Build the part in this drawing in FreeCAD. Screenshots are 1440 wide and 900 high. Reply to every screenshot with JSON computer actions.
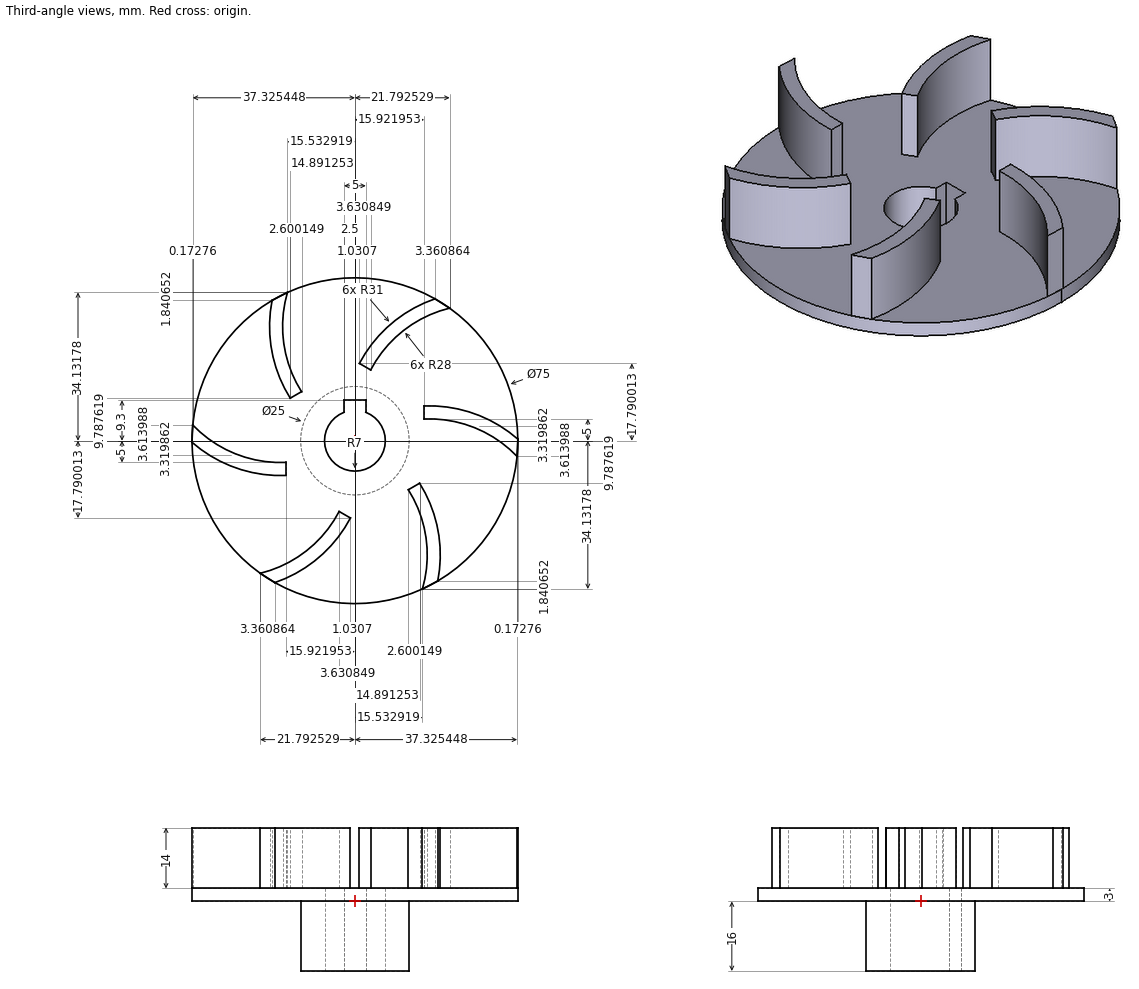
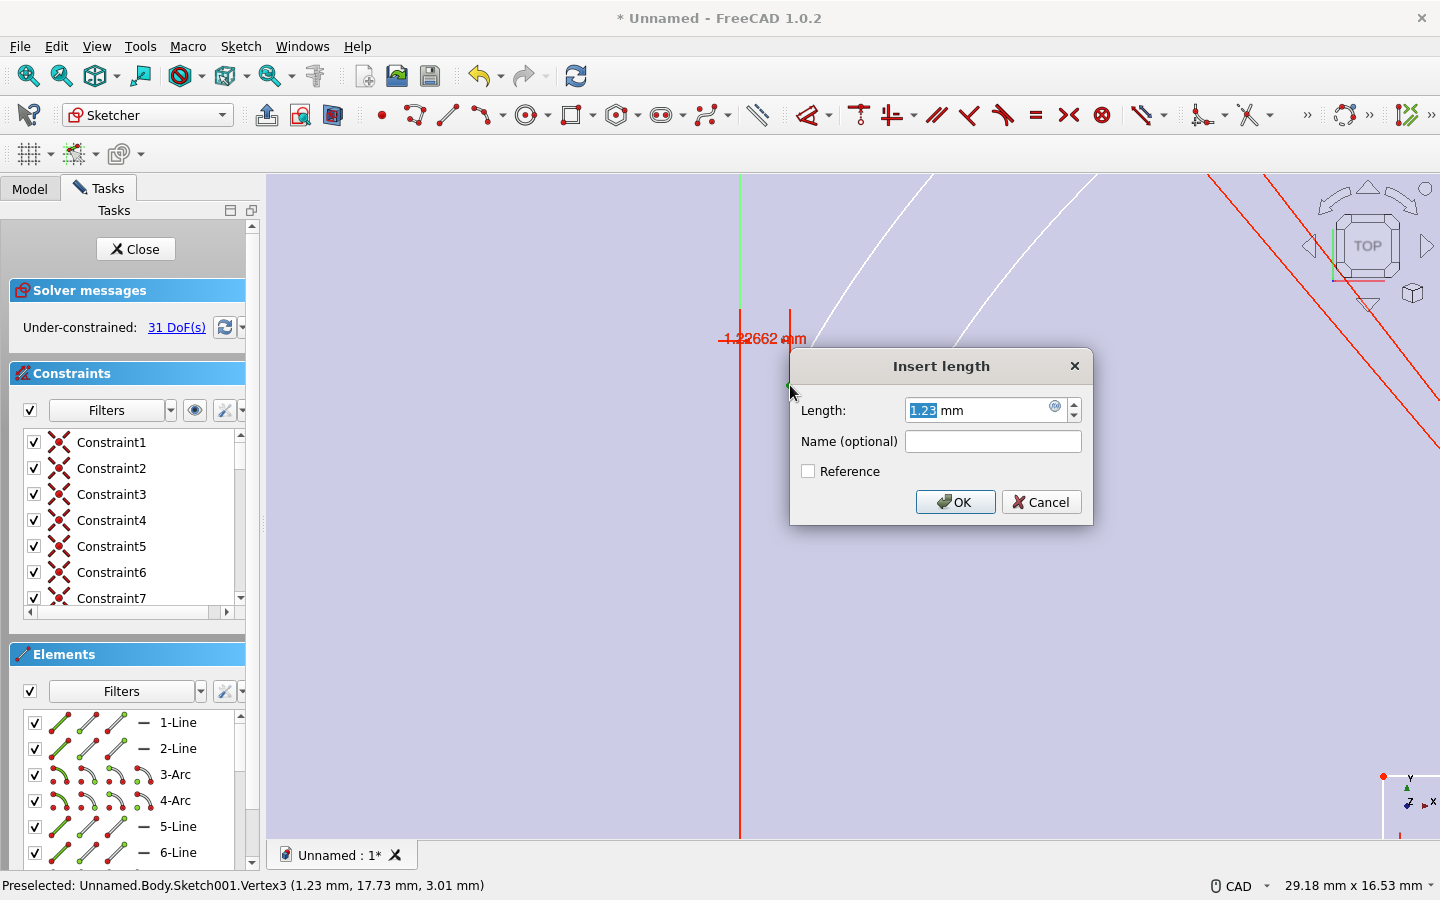
{"action": "type", "text": "1.0307"}
{"action": "key", "text": "Return"}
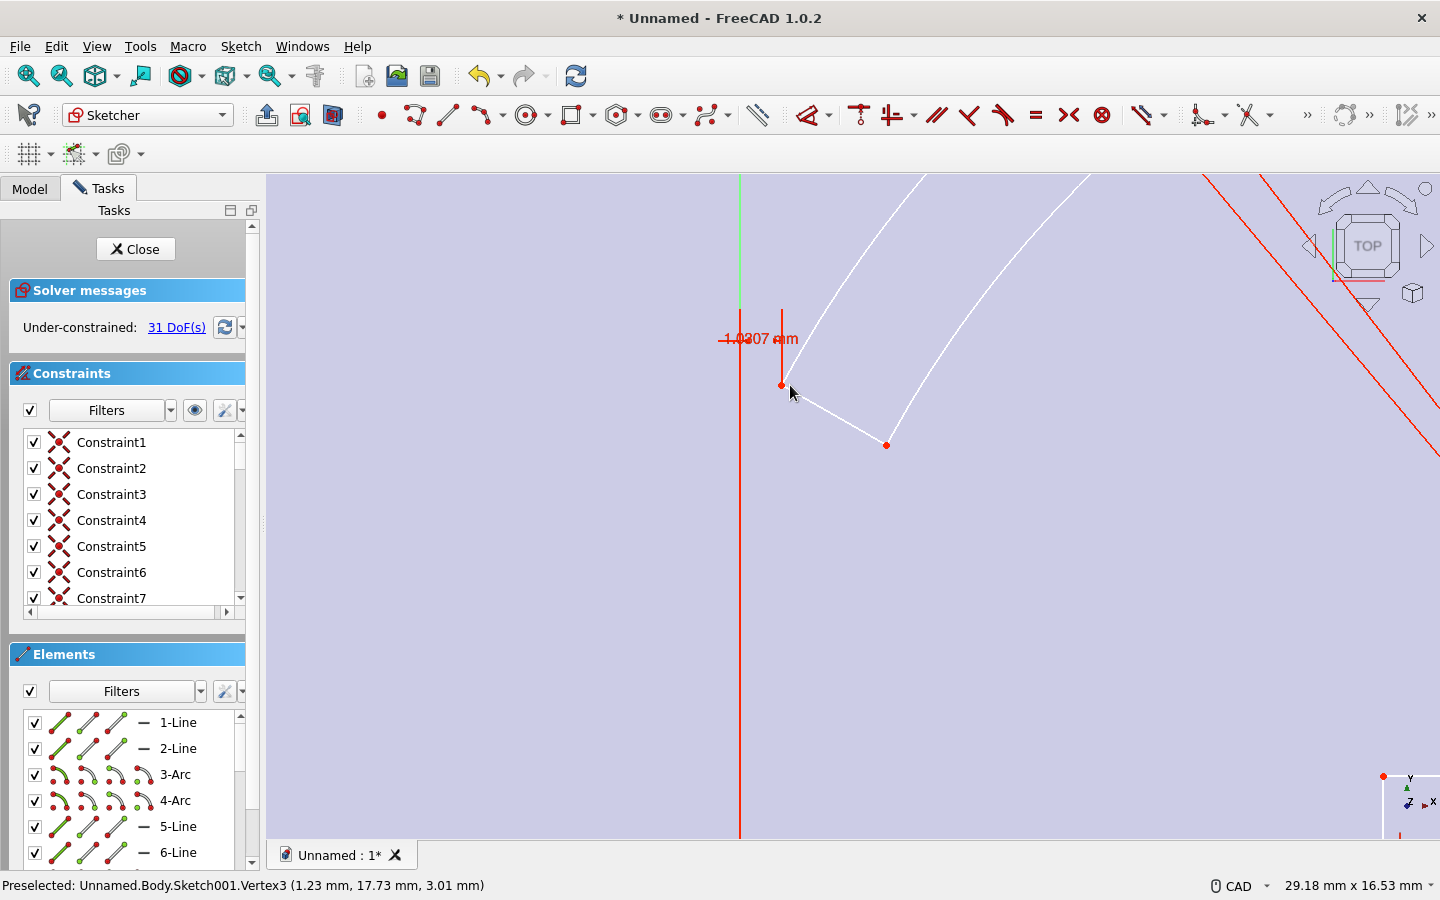
{"action": "scroll", "coordinate": [793, 389], "scroll_direction": "down", "scroll_amount": 9}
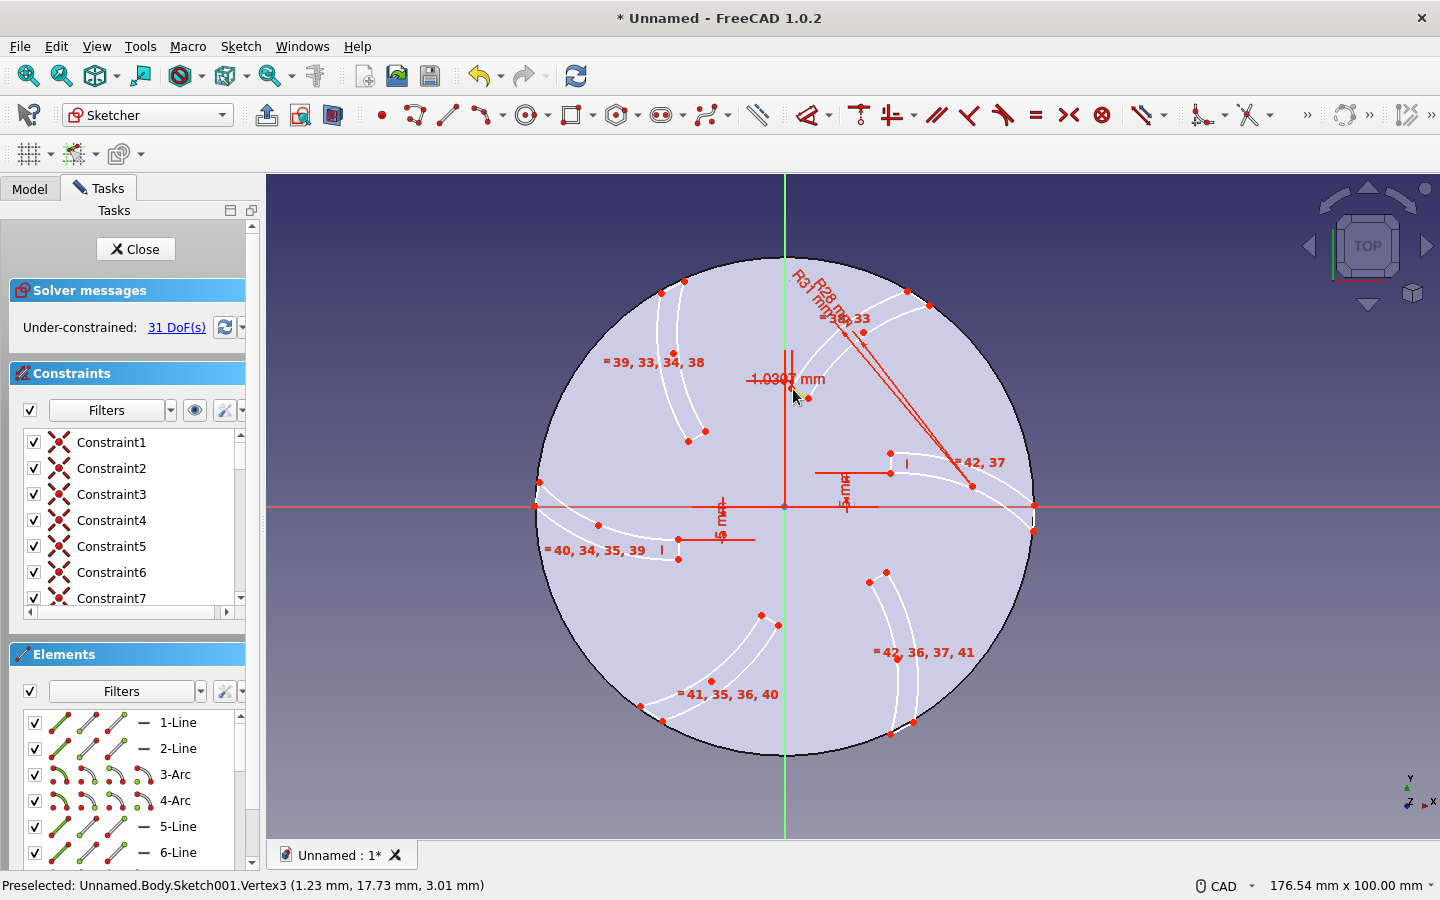
{"action": "scroll", "coordinate": [779, 625], "scroll_direction": "up", "scroll_amount": 9}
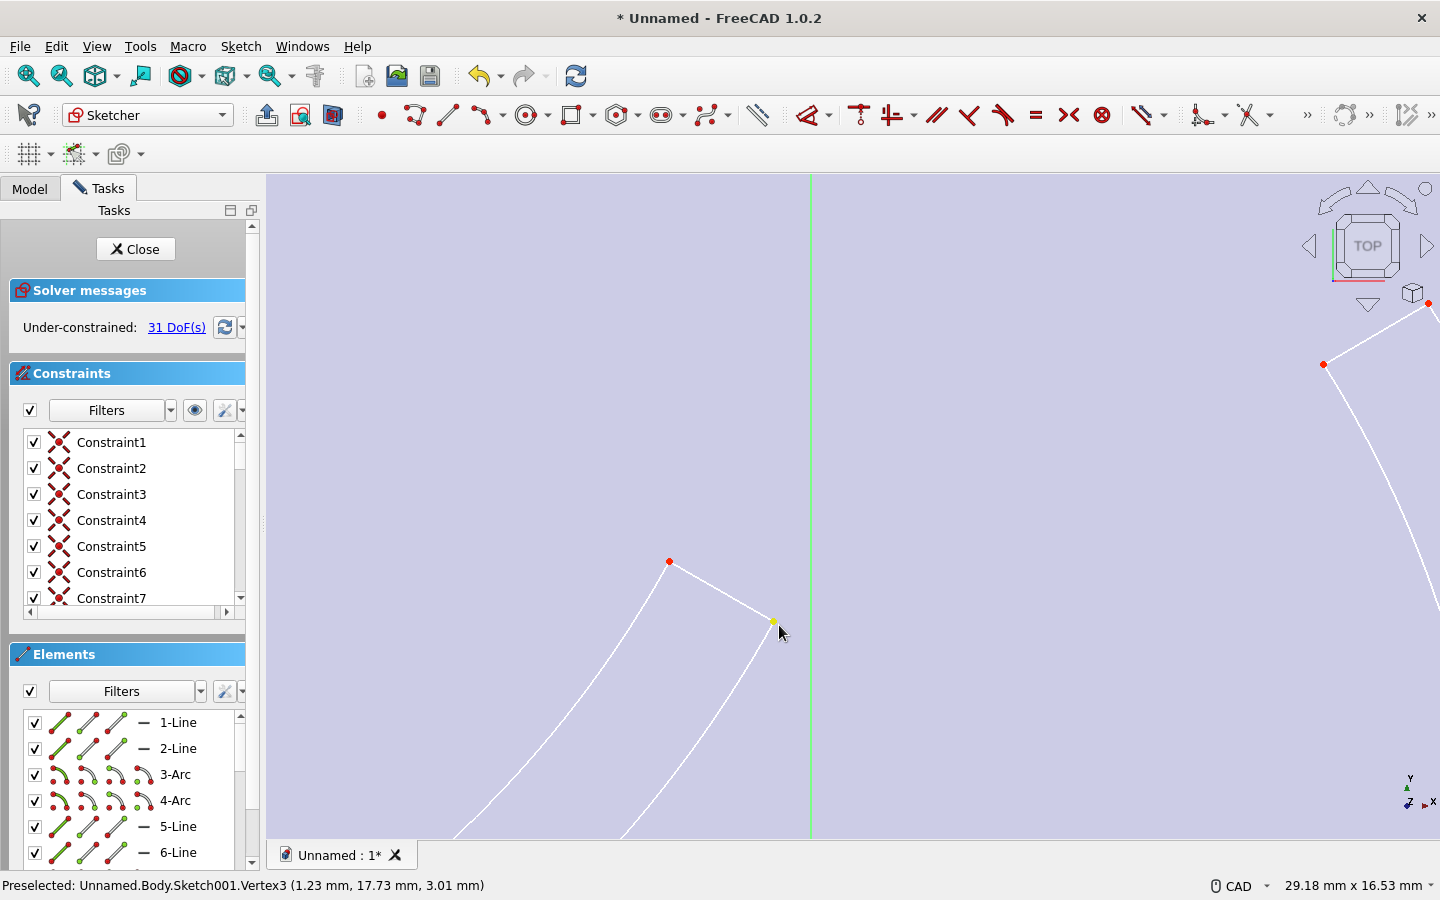
{"action": "left_click", "coordinate": [774, 622]}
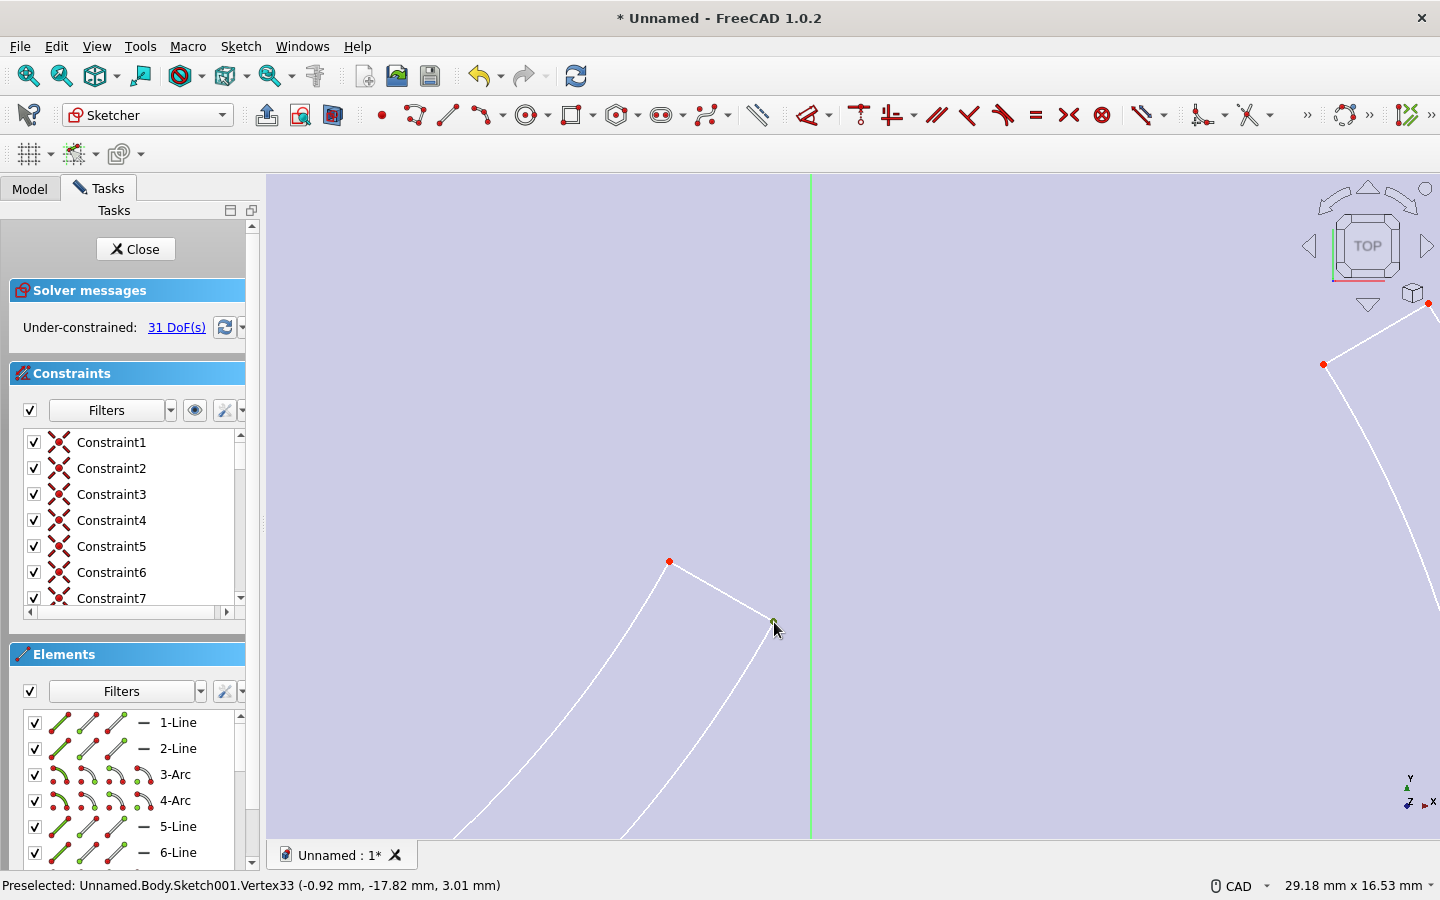
{"action": "key", "text": "l"}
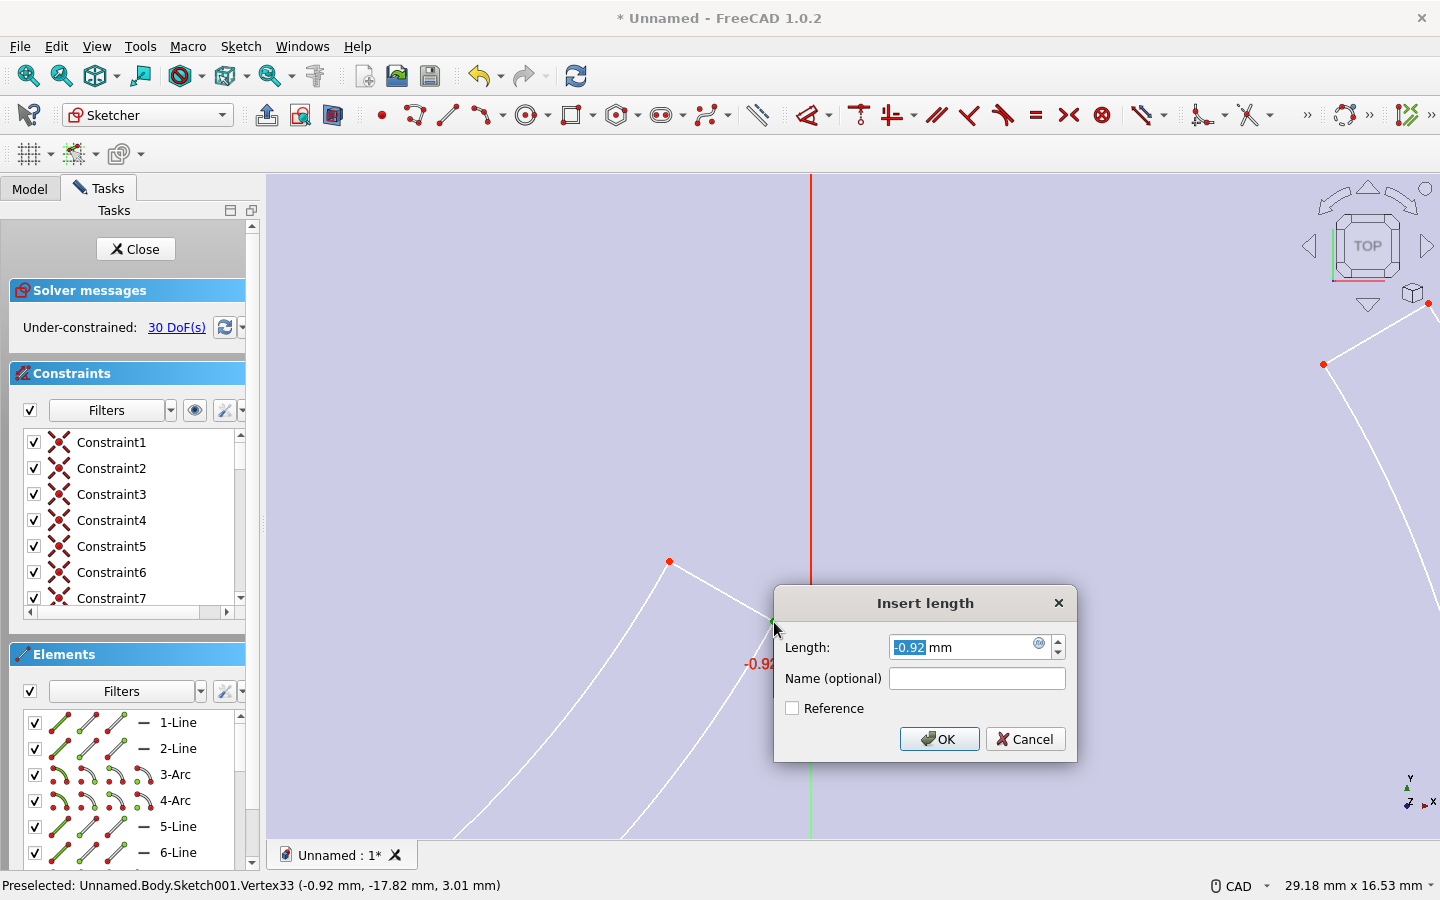
{"action": "type", "text": "-1.0307"}
{"action": "key", "text": "Return"}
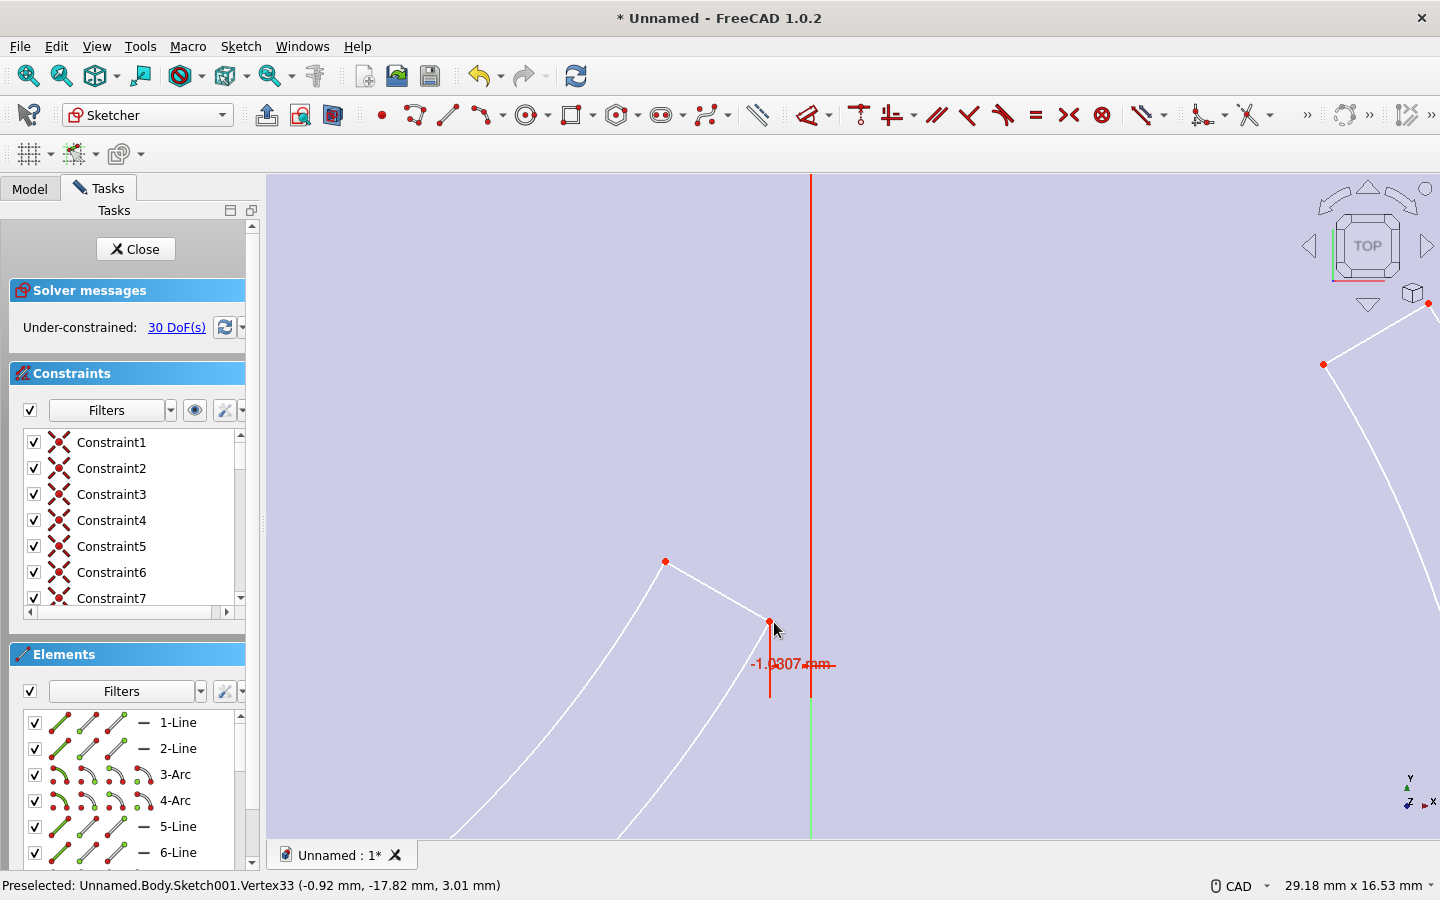
{"action": "scroll", "coordinate": [779, 626], "scroll_direction": "down", "scroll_amount": 9}